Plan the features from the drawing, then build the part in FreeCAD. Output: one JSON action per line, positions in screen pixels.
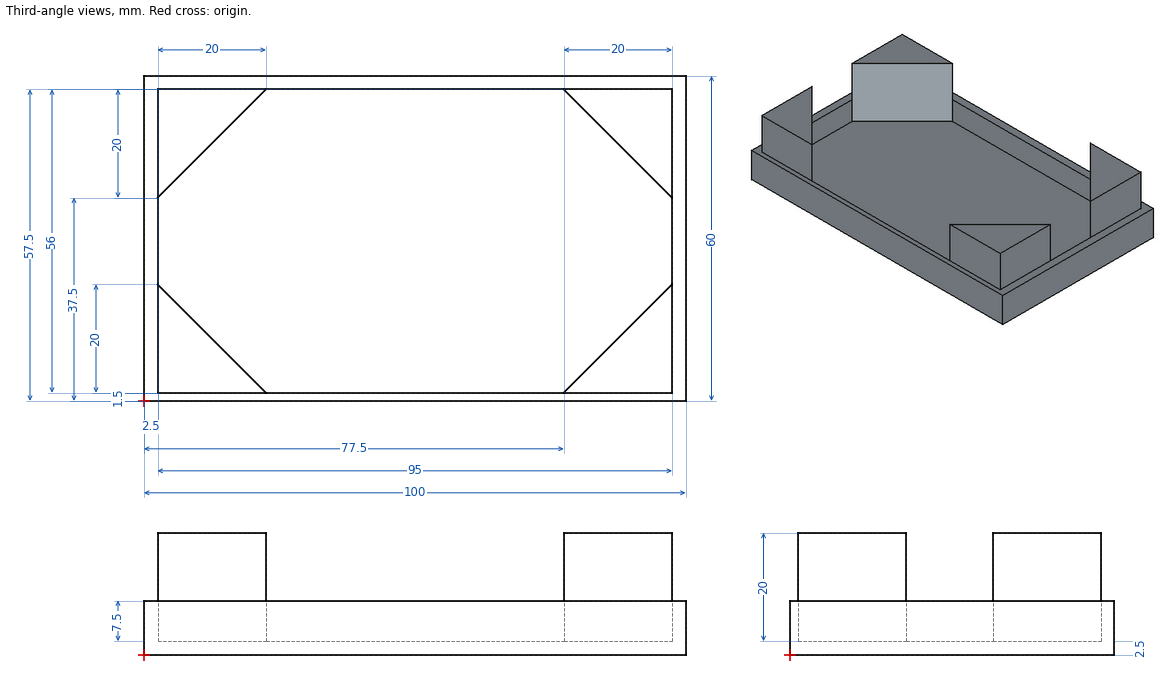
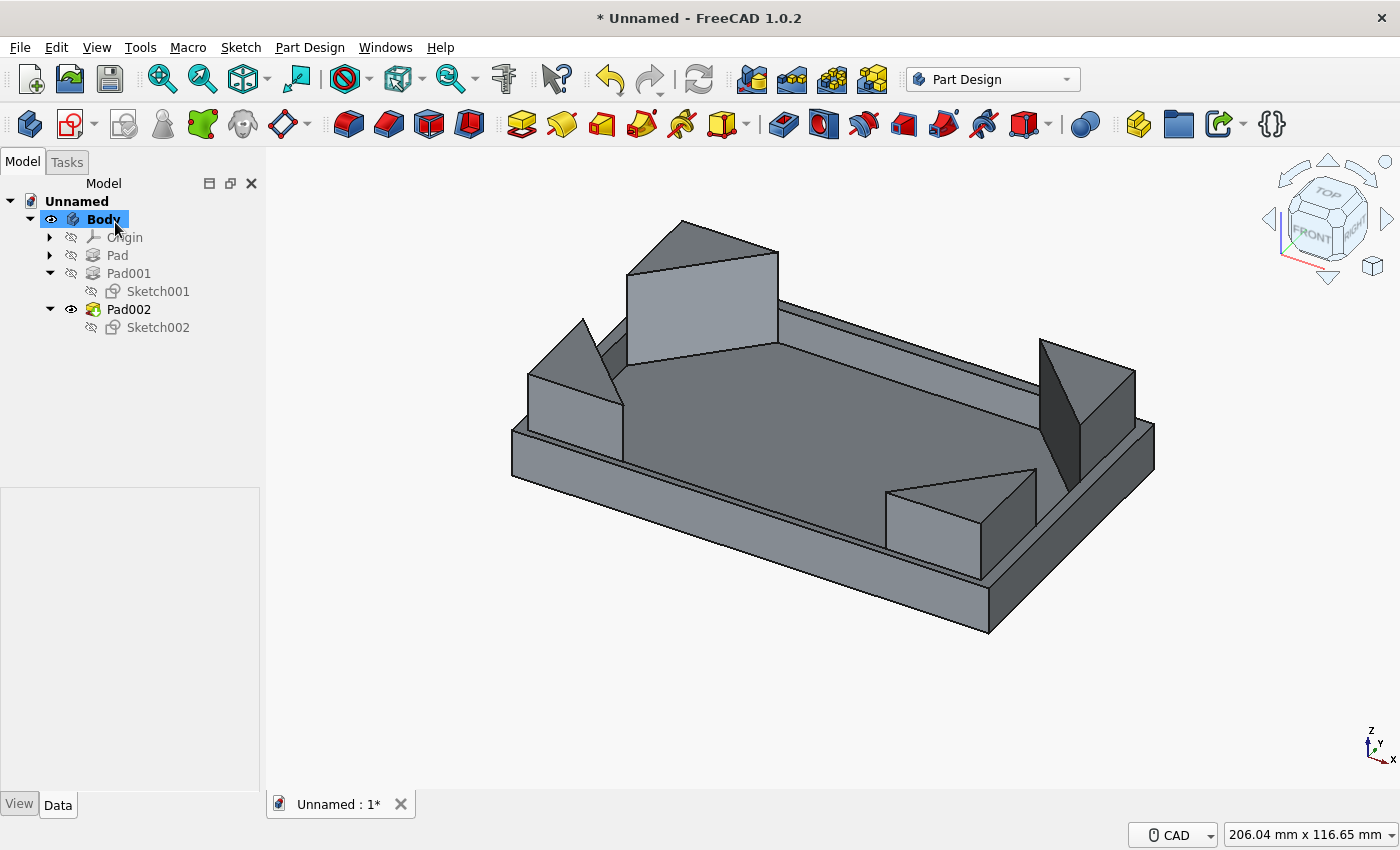
{"action": "key", "text": "0"}